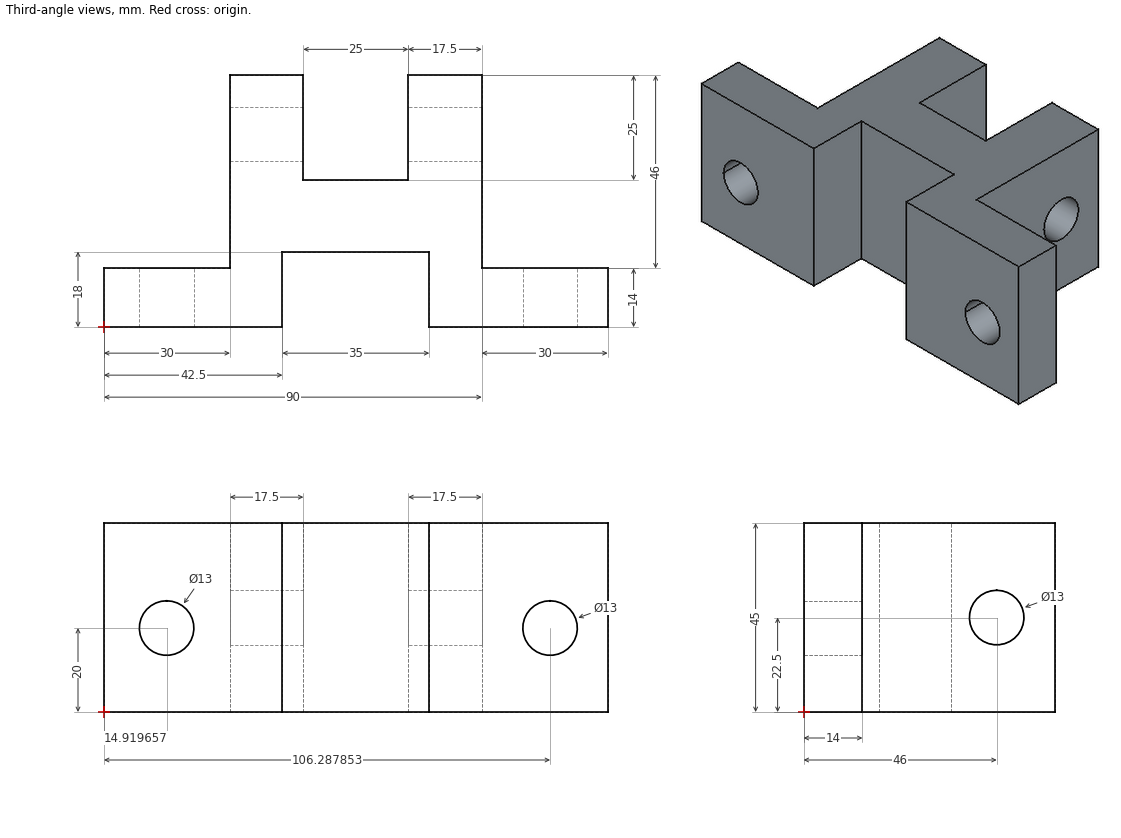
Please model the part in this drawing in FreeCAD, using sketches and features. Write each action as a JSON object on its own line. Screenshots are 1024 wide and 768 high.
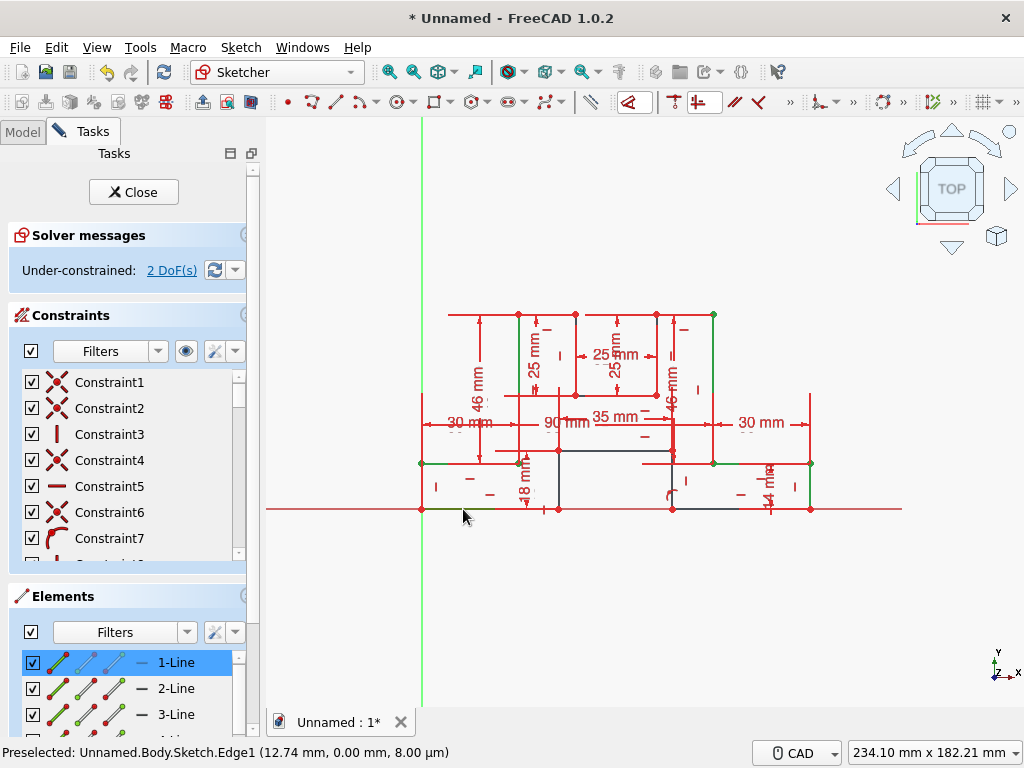
{"action": "key", "text": "l"}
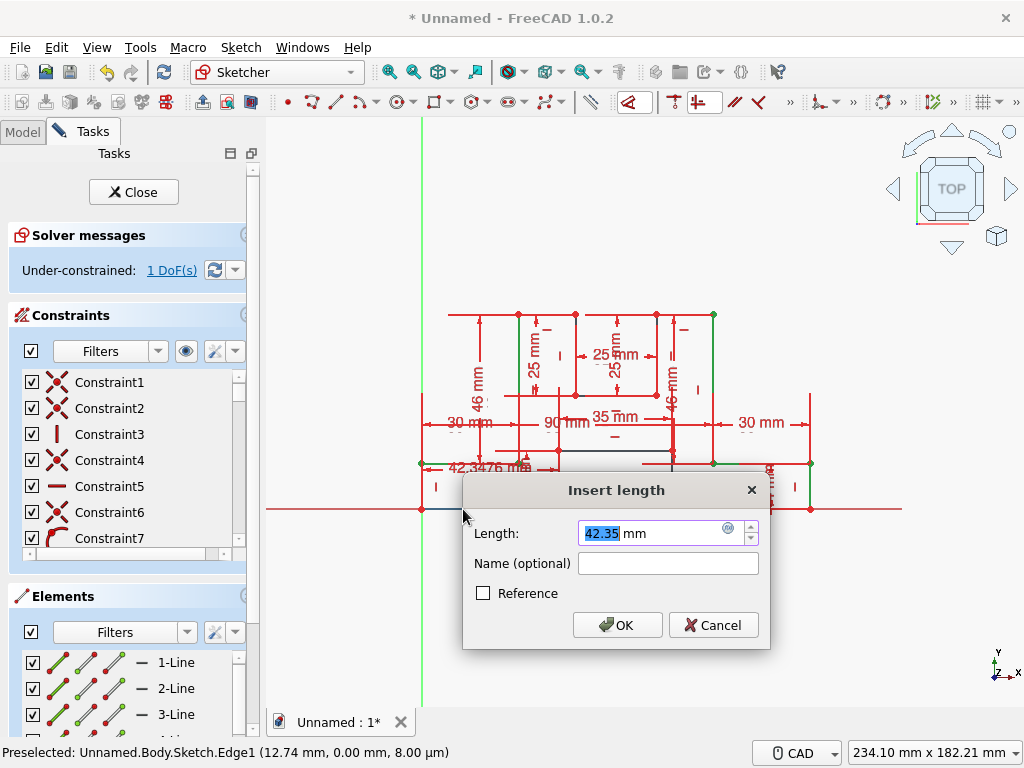
{"action": "type", "text": "42.5"}
{"action": "key", "text": "Return"}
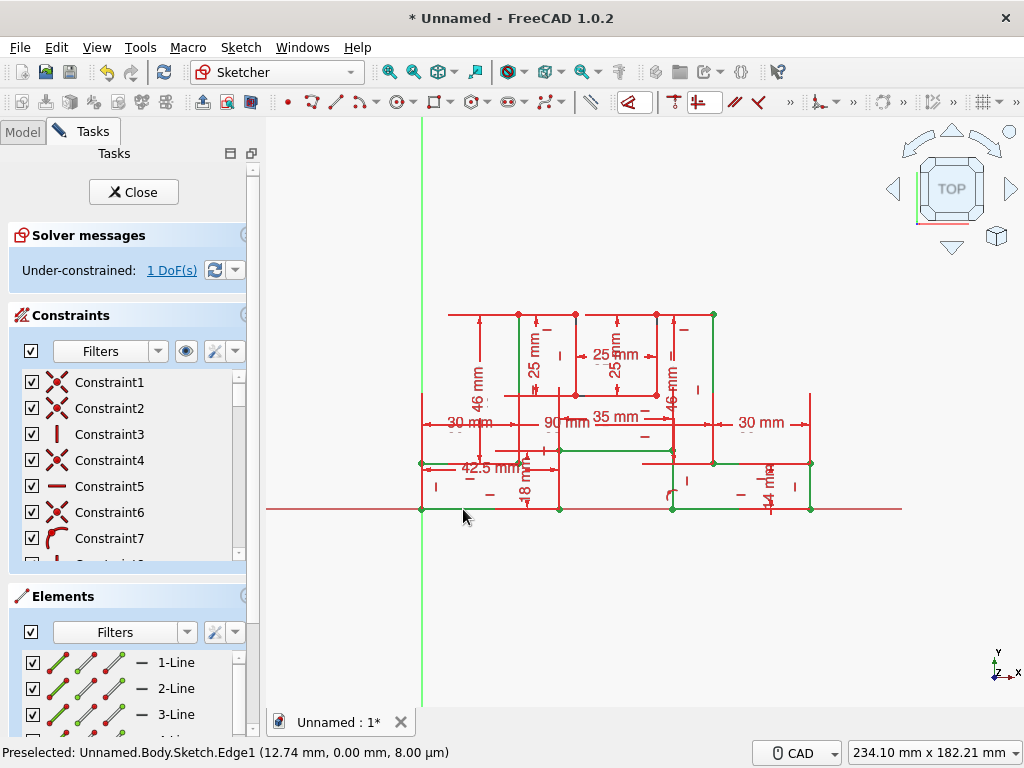
{"action": "left_click", "coordinate": [696, 315]}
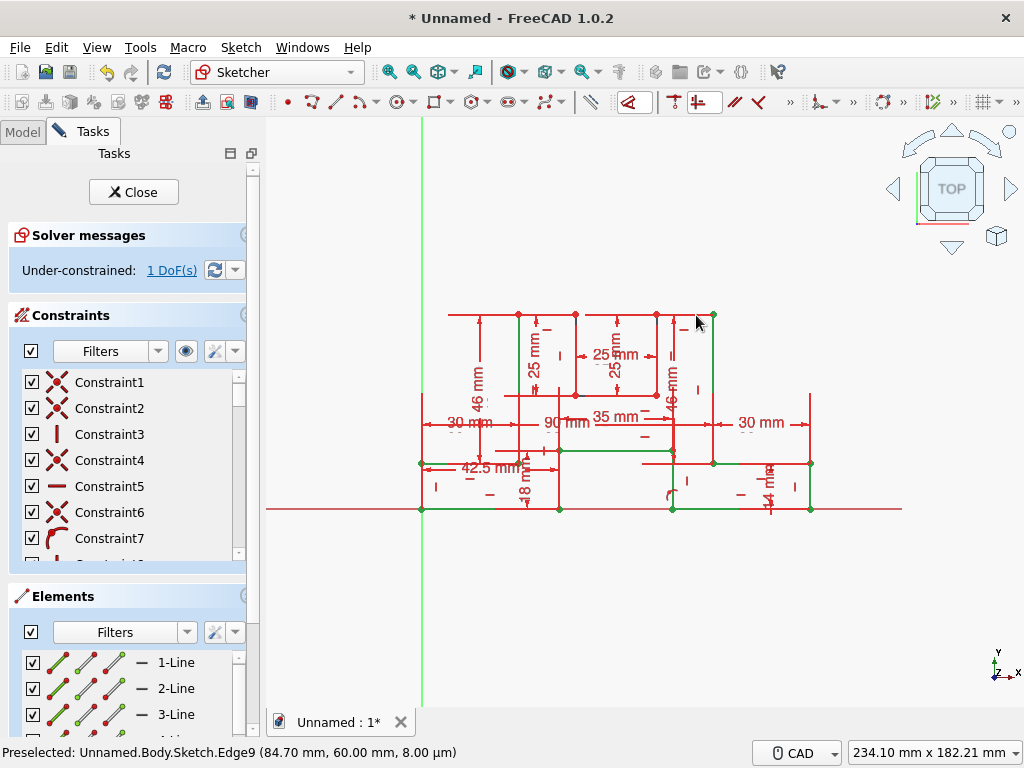
{"action": "key", "text": "l"}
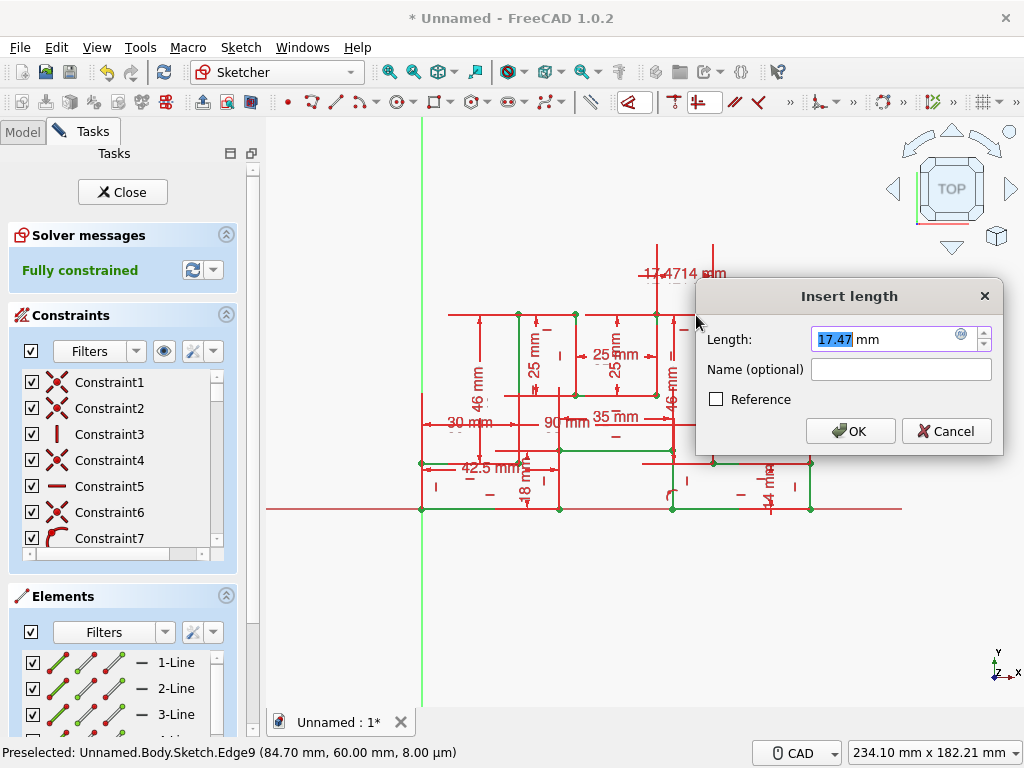
{"action": "type", "text": "17.5"}
{"action": "key", "text": "Return"}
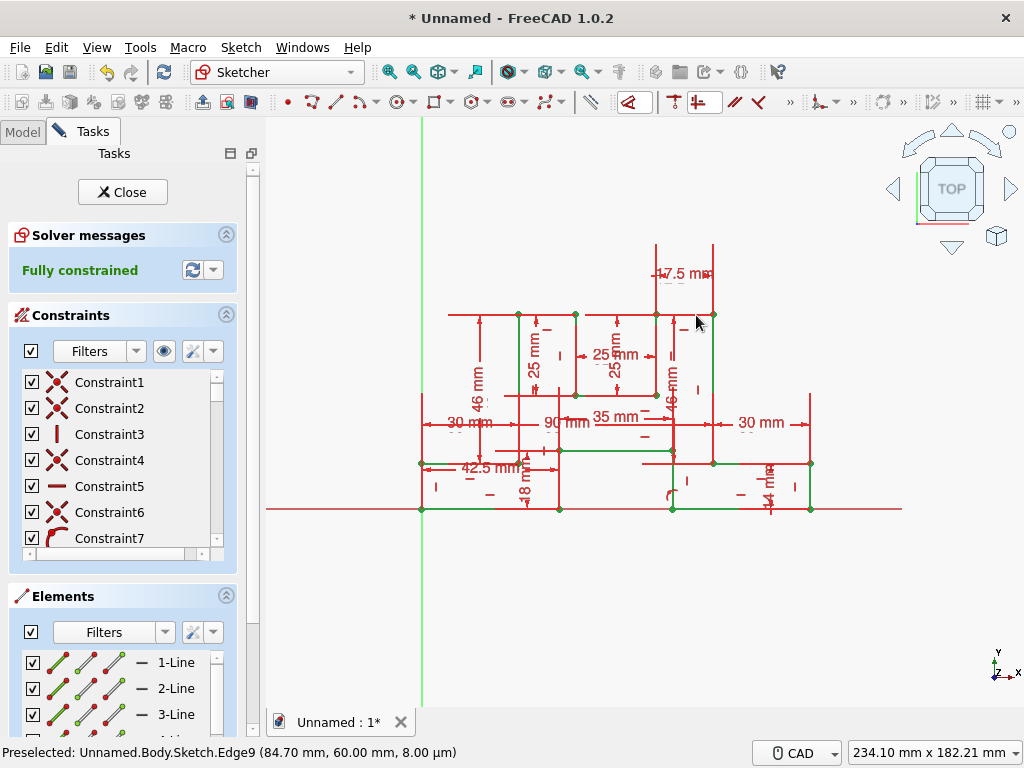
{"action": "left_click", "coordinate": [123, 192]}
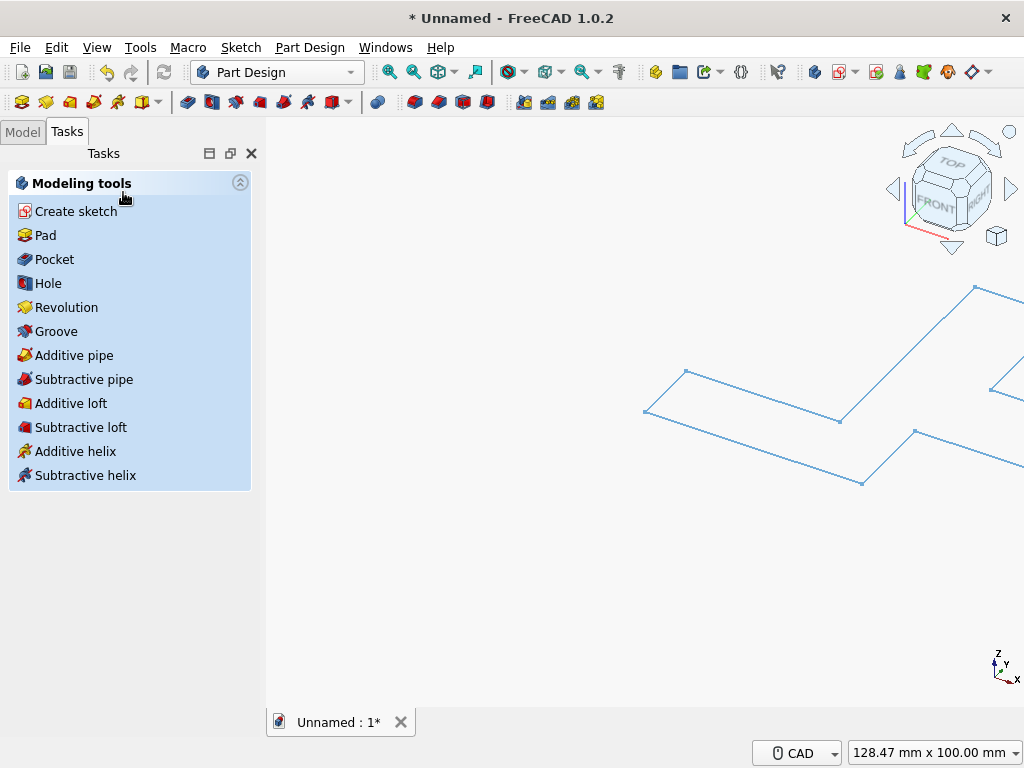
{"action": "left_click", "coordinate": [22, 102]}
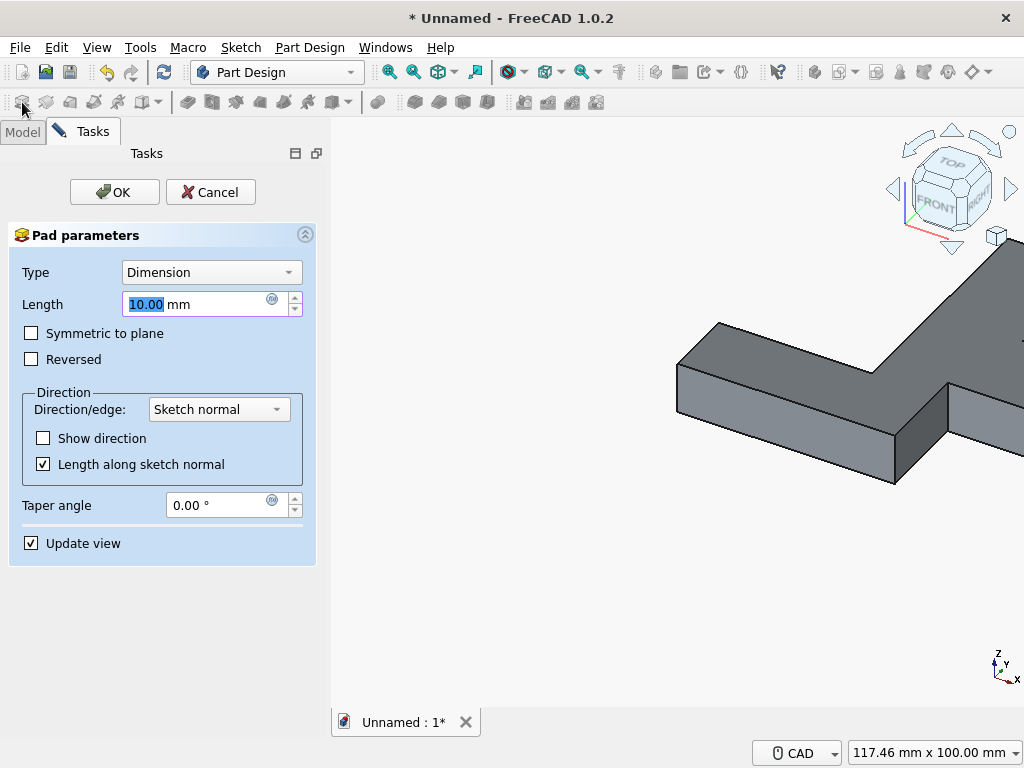
{"action": "type", "text": "45"}
{"action": "key", "text": "Tab"}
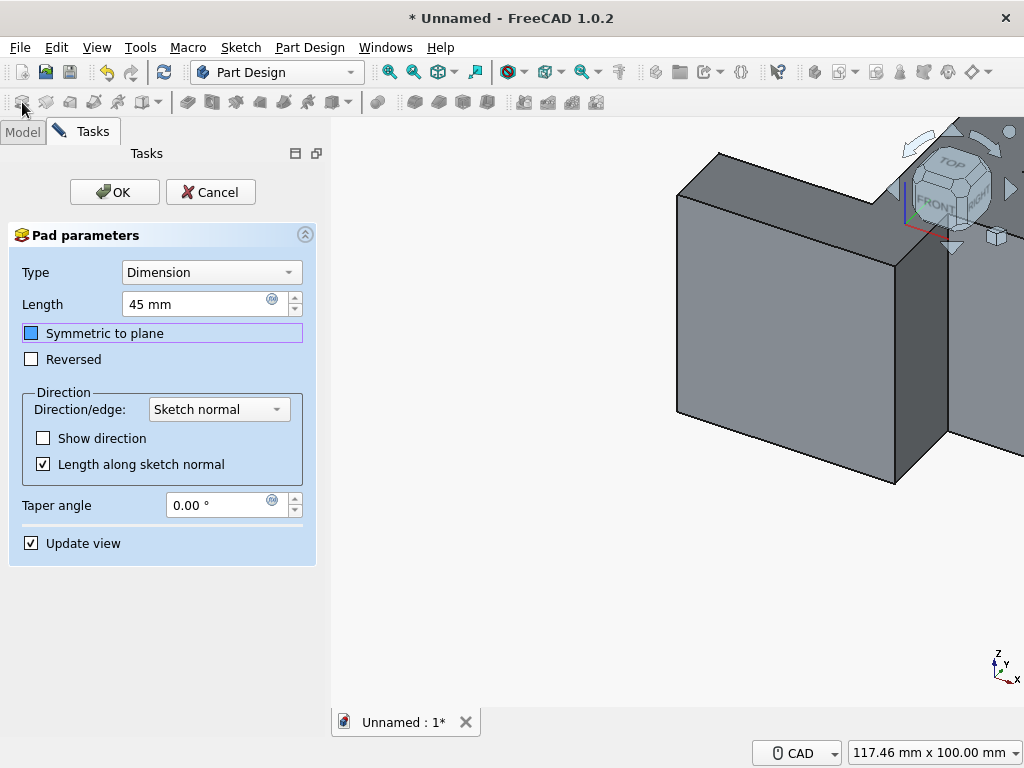
{"action": "left_click", "coordinate": [115, 192]}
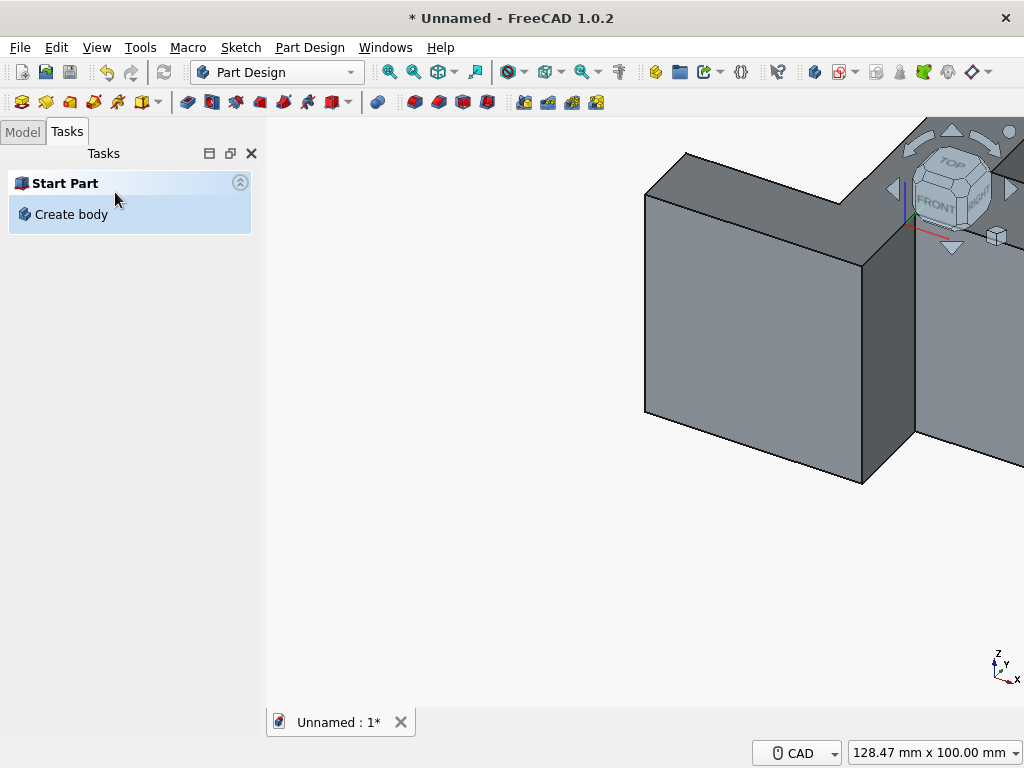
{"action": "left_click", "coordinate": [390, 72]}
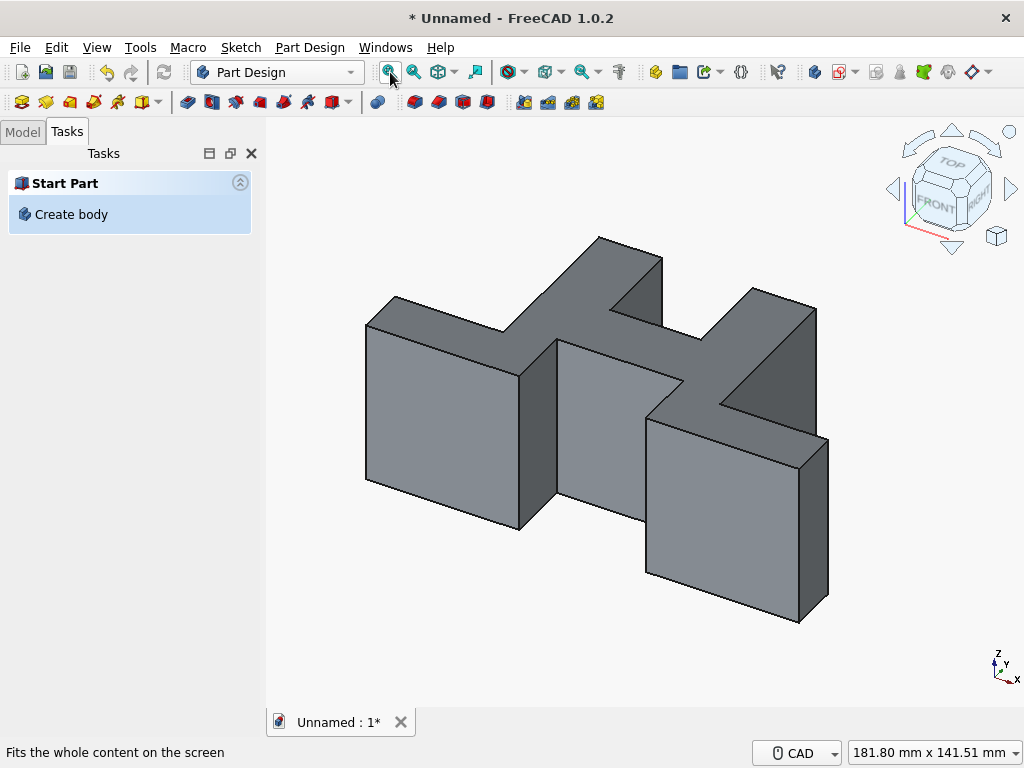
{"action": "key", "text": "6"}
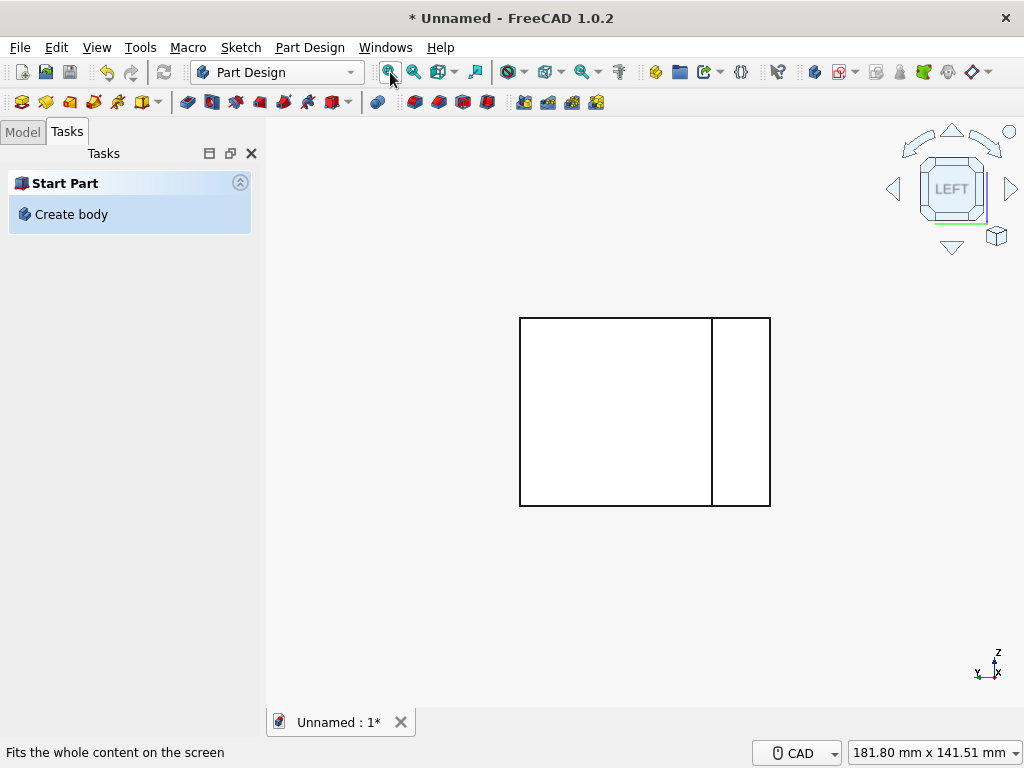
{"action": "left_click", "coordinate": [390, 72]}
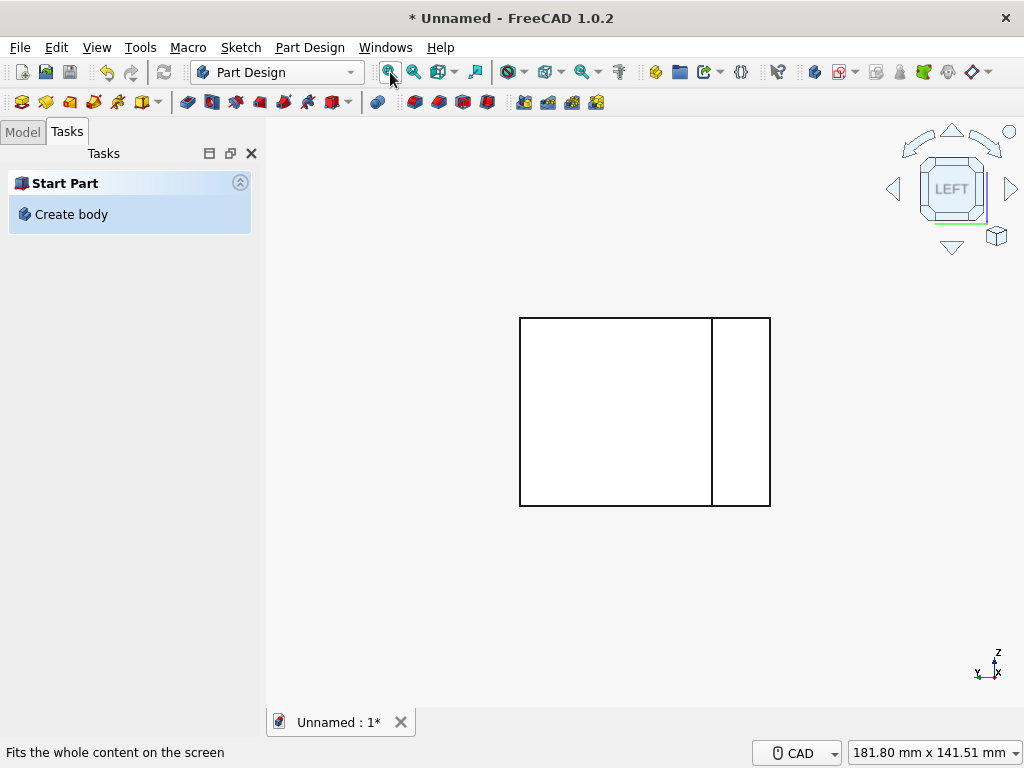
{"action": "left_click", "coordinate": [616, 411]}